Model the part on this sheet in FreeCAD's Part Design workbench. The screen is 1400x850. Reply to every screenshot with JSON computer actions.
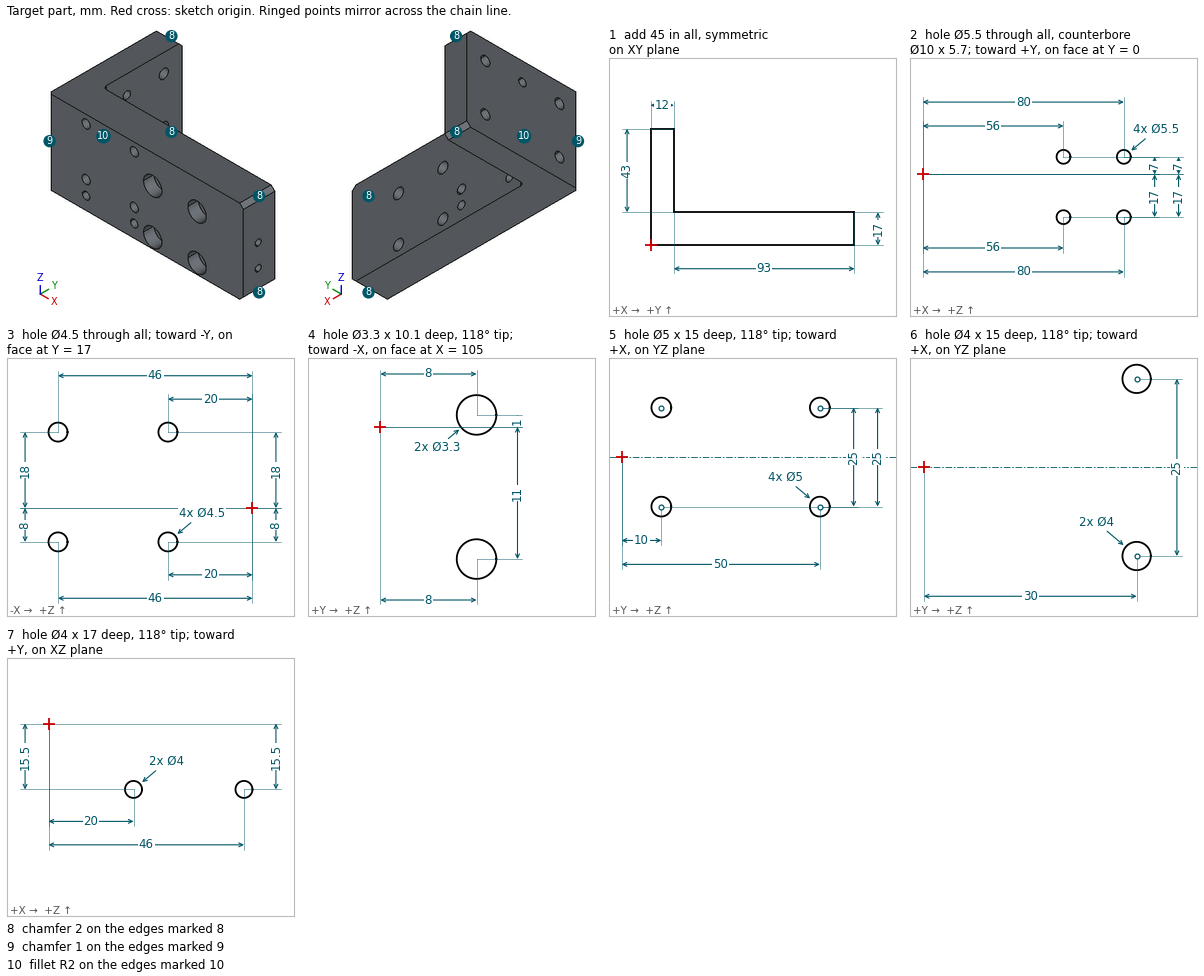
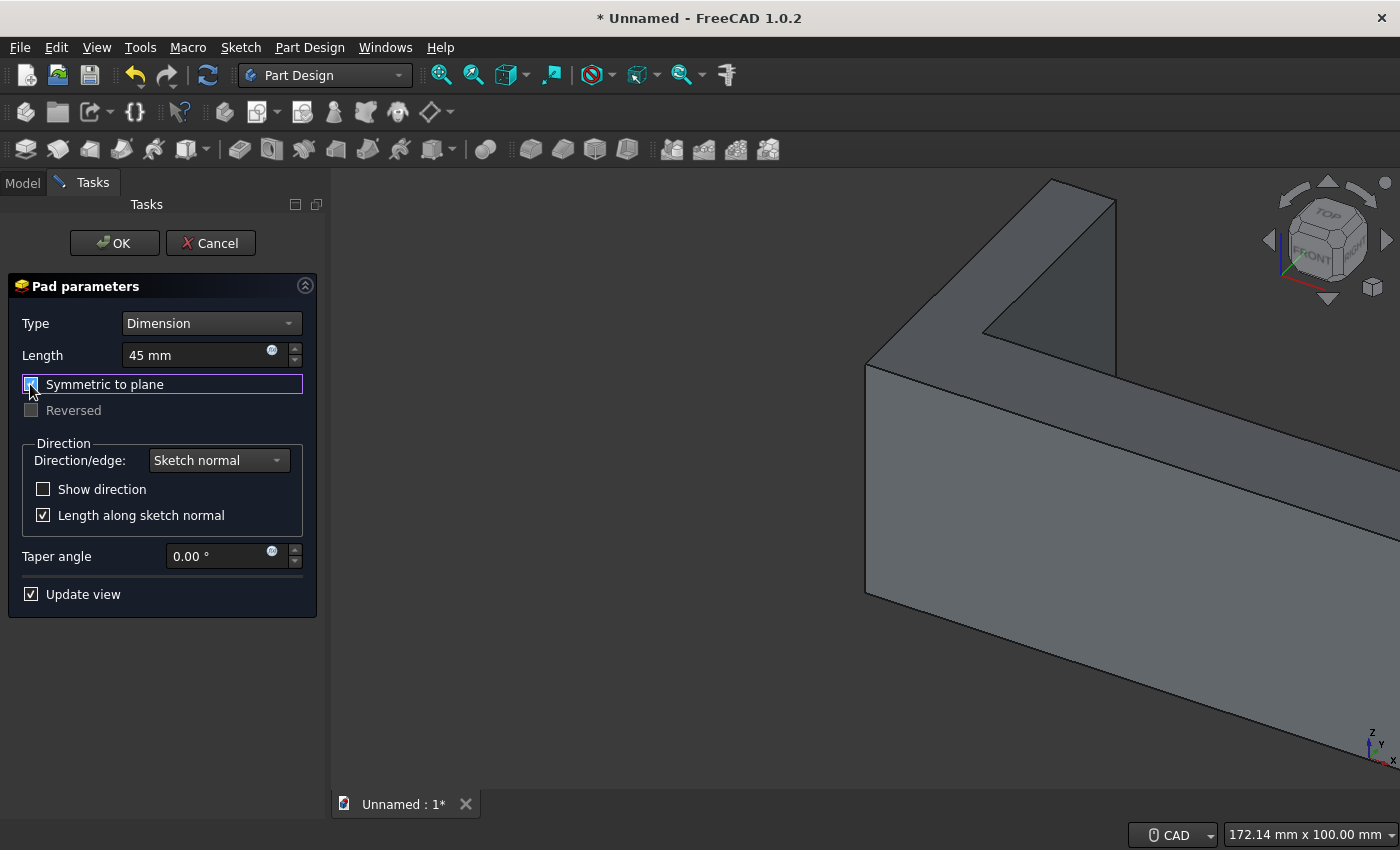
{"action": "left_click", "coordinate": [115, 243]}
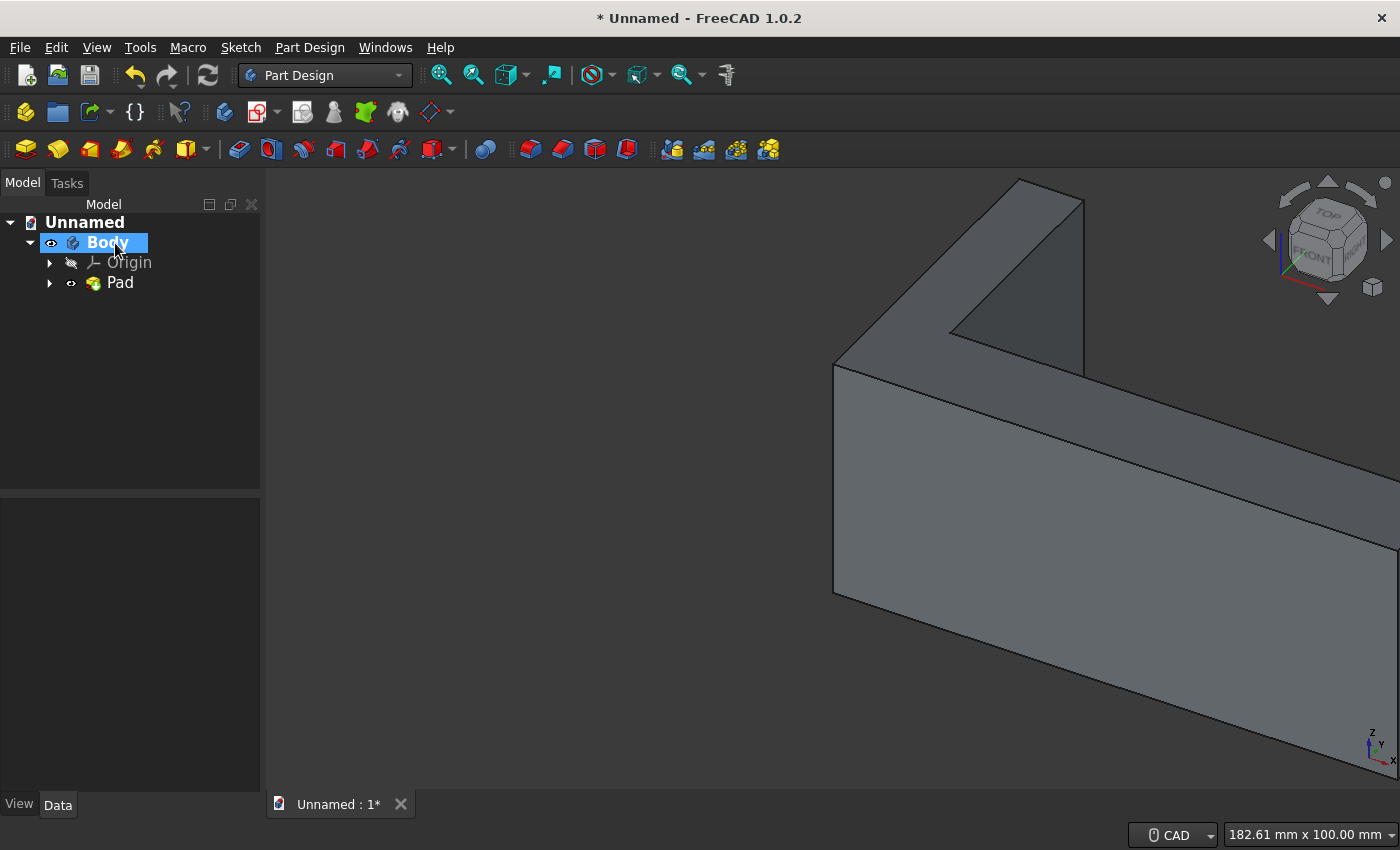
{"action": "left_click", "coordinate": [442, 76]}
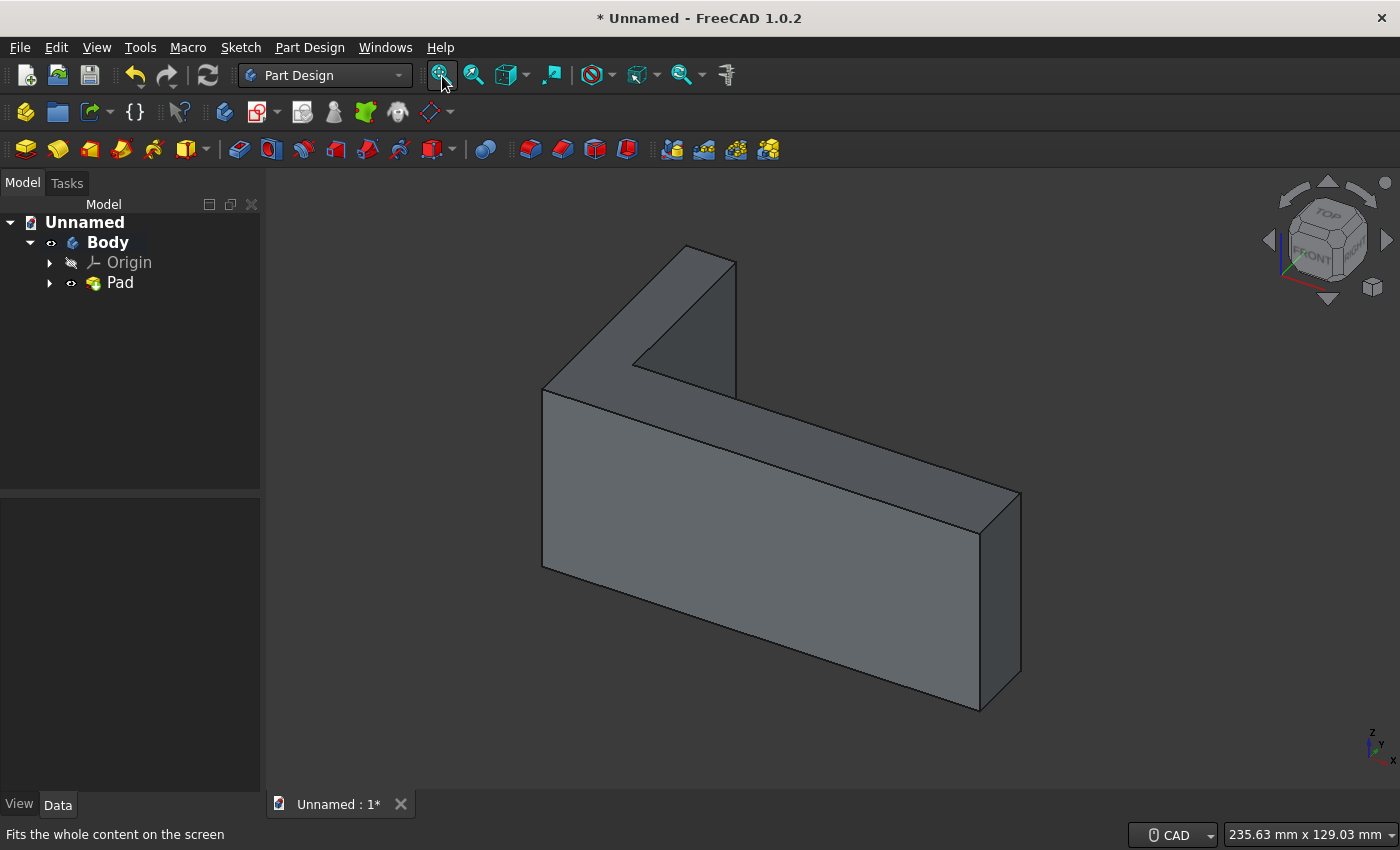
{"action": "left_click", "coordinate": [886, 591]}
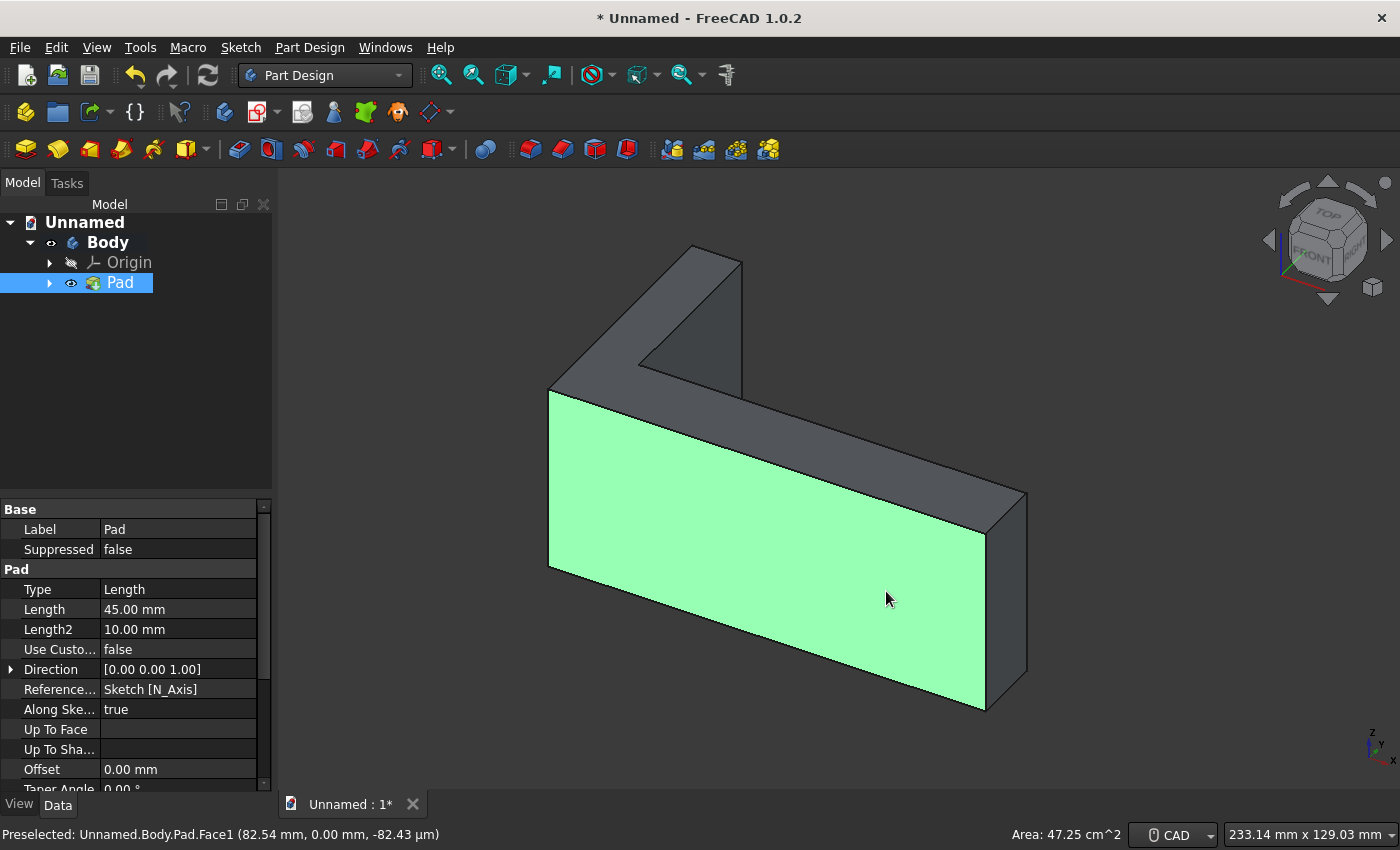
{"action": "left_click", "coordinate": [258, 112]}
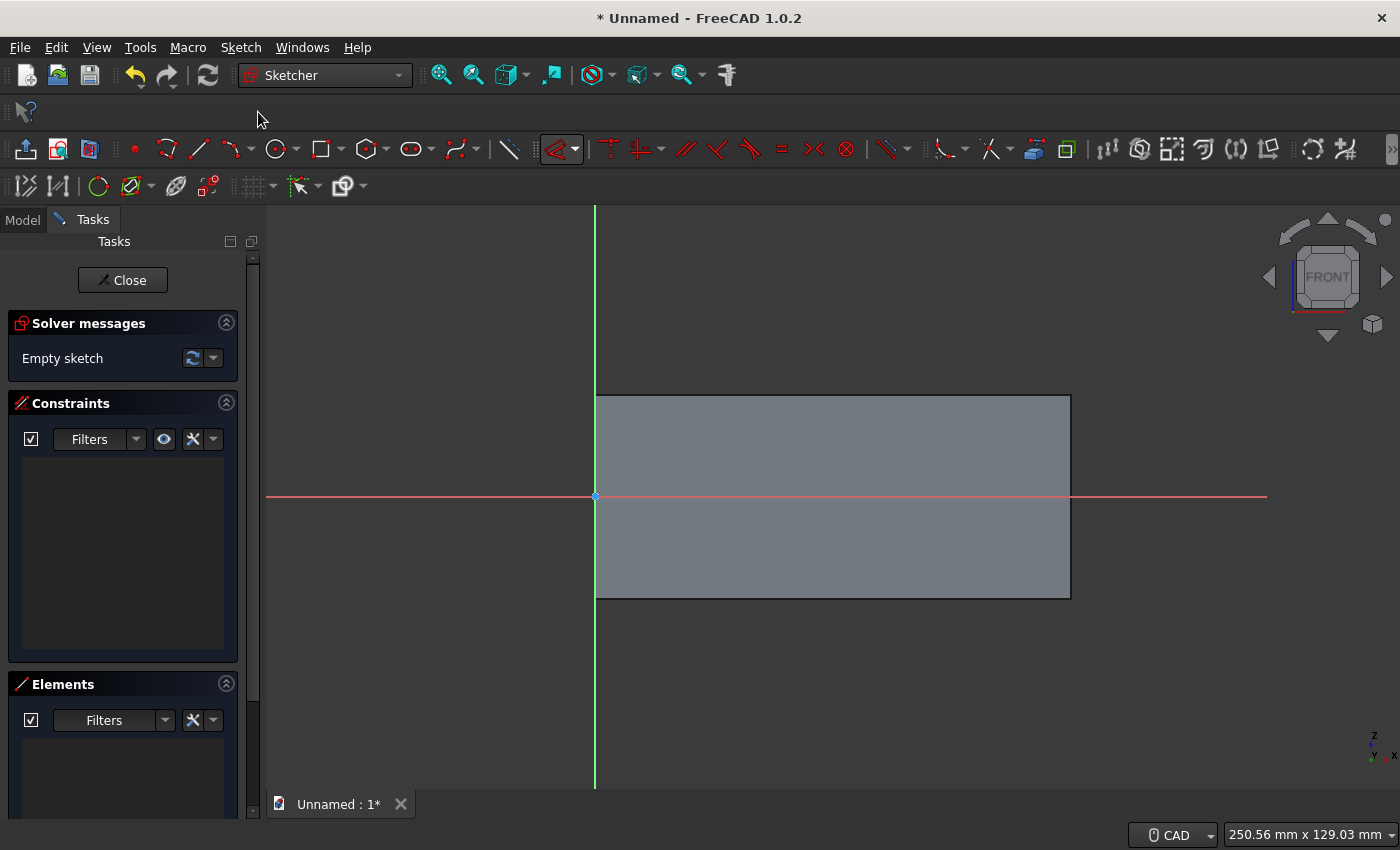
{"action": "scroll", "coordinate": [984, 533], "scroll_direction": "up", "scroll_amount": 5}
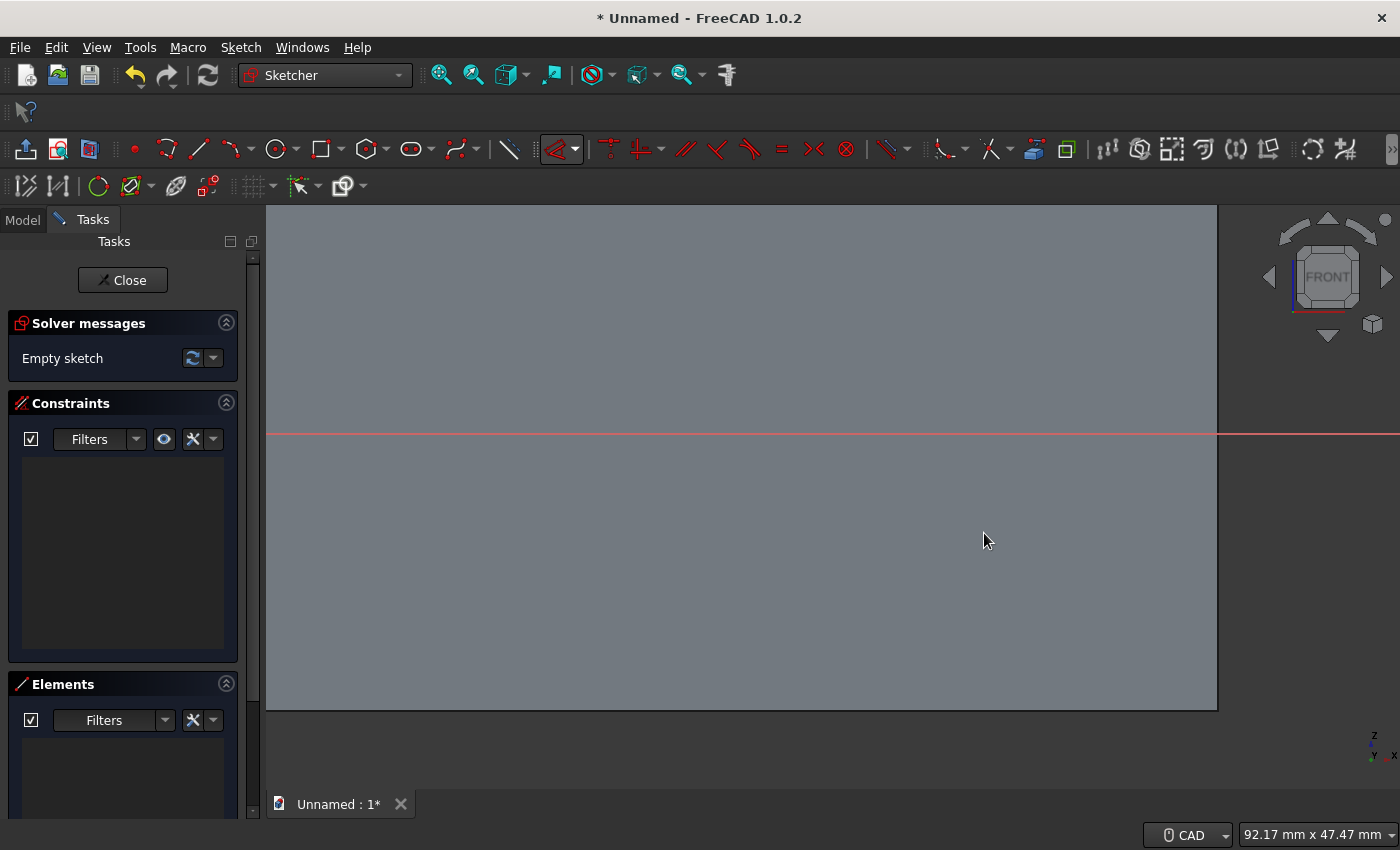
{"action": "key", "text": "g c"}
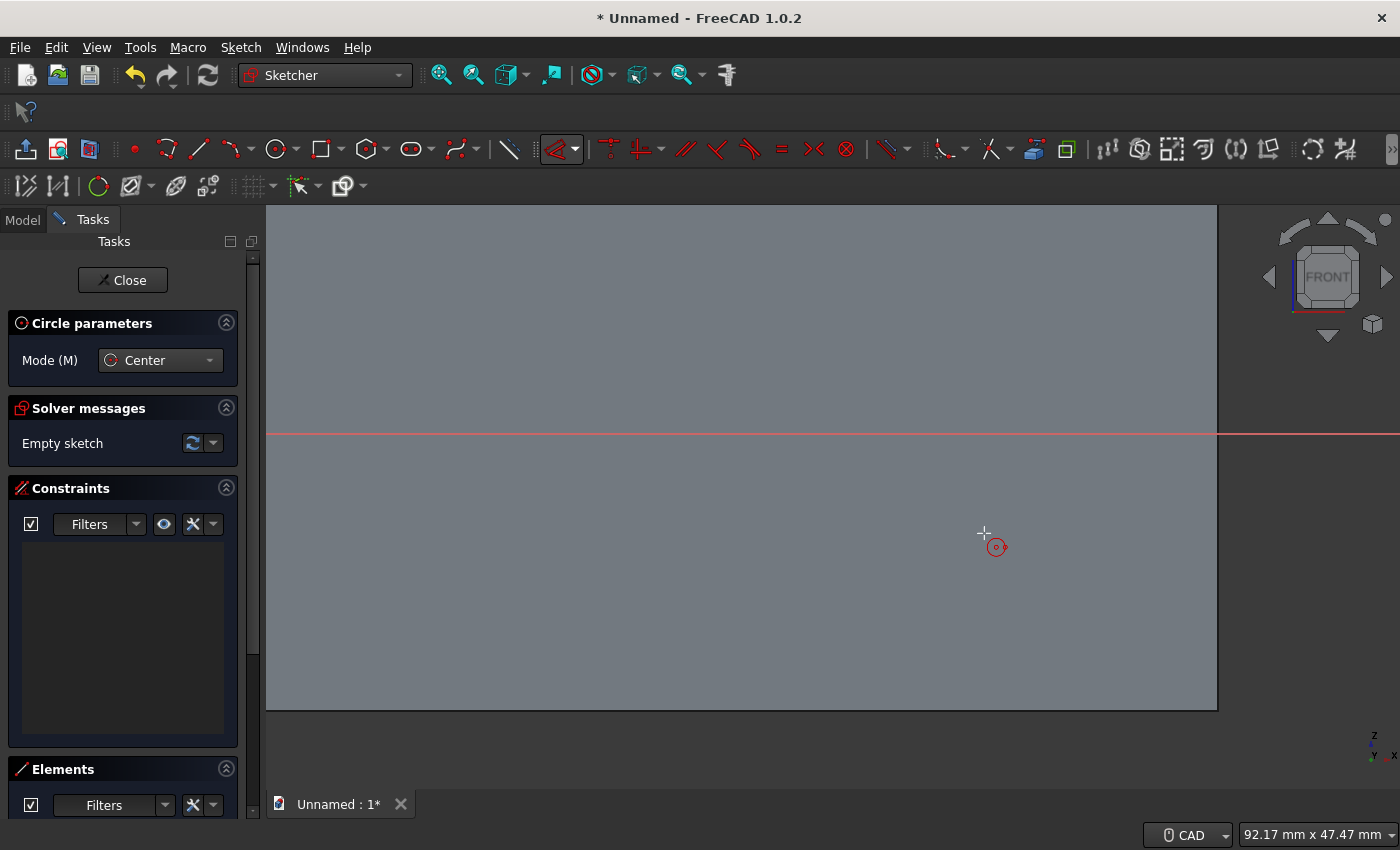
{"action": "left_click", "coordinate": [911, 348]}
{"action": "left_click", "coordinate": [935, 324]}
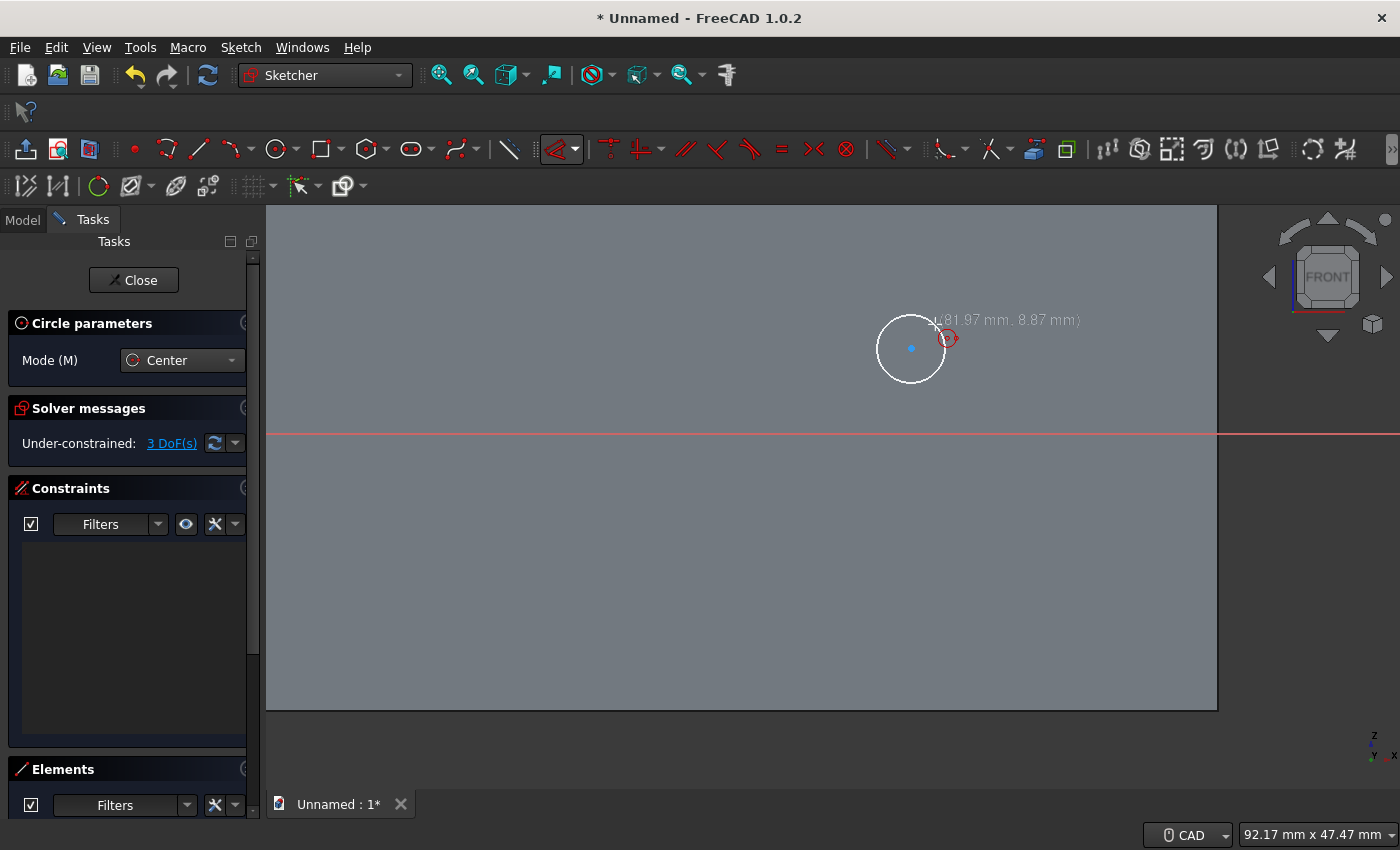
{"action": "left_click", "coordinate": [616, 348]}
{"action": "left_click", "coordinate": [639, 324]}